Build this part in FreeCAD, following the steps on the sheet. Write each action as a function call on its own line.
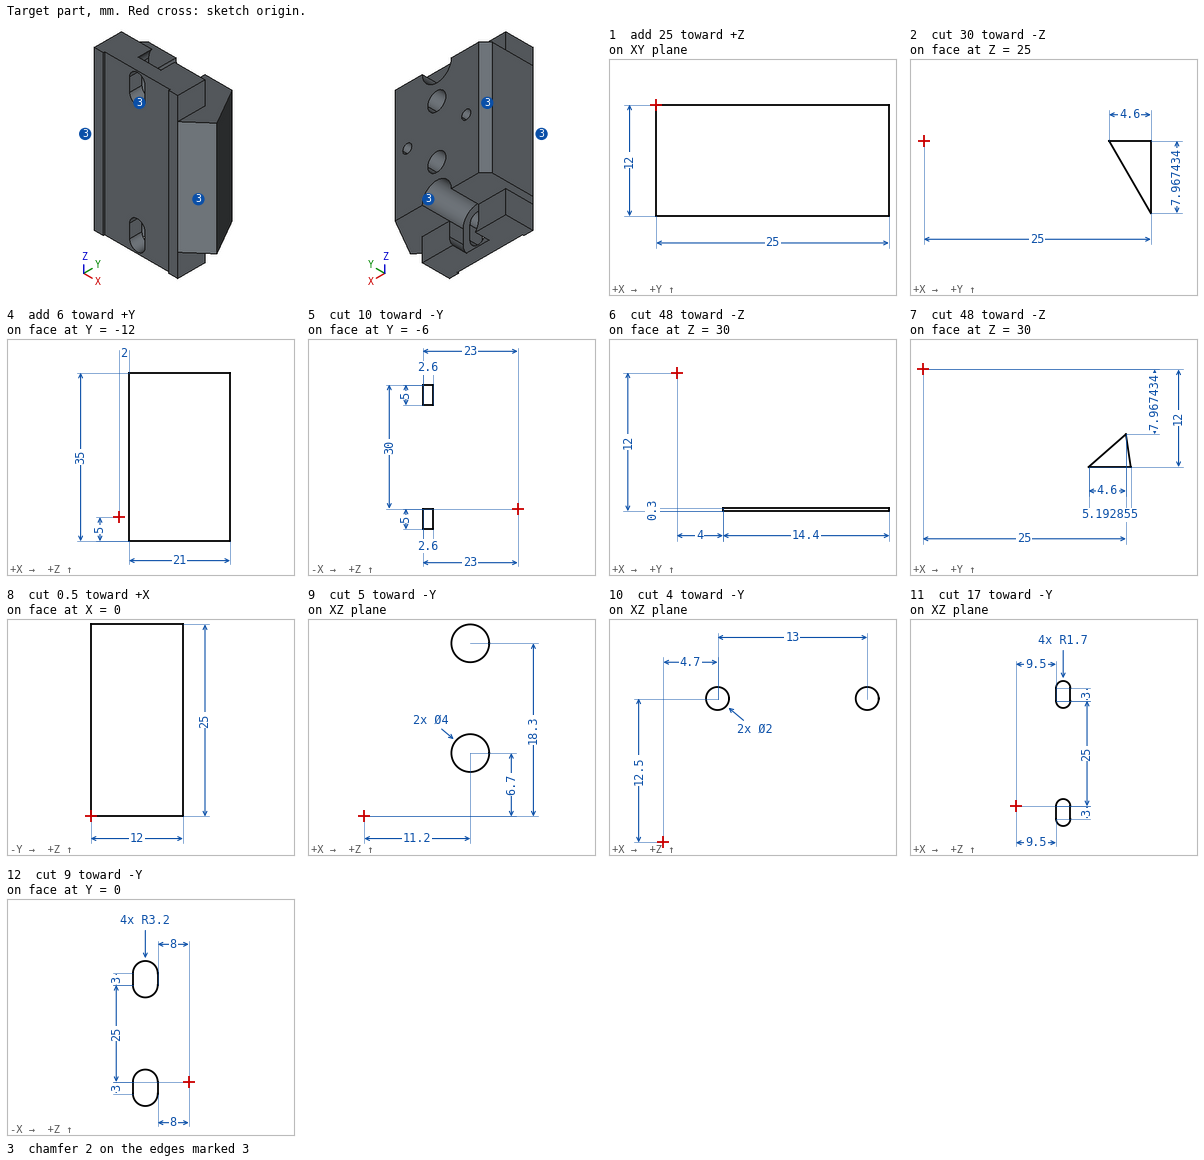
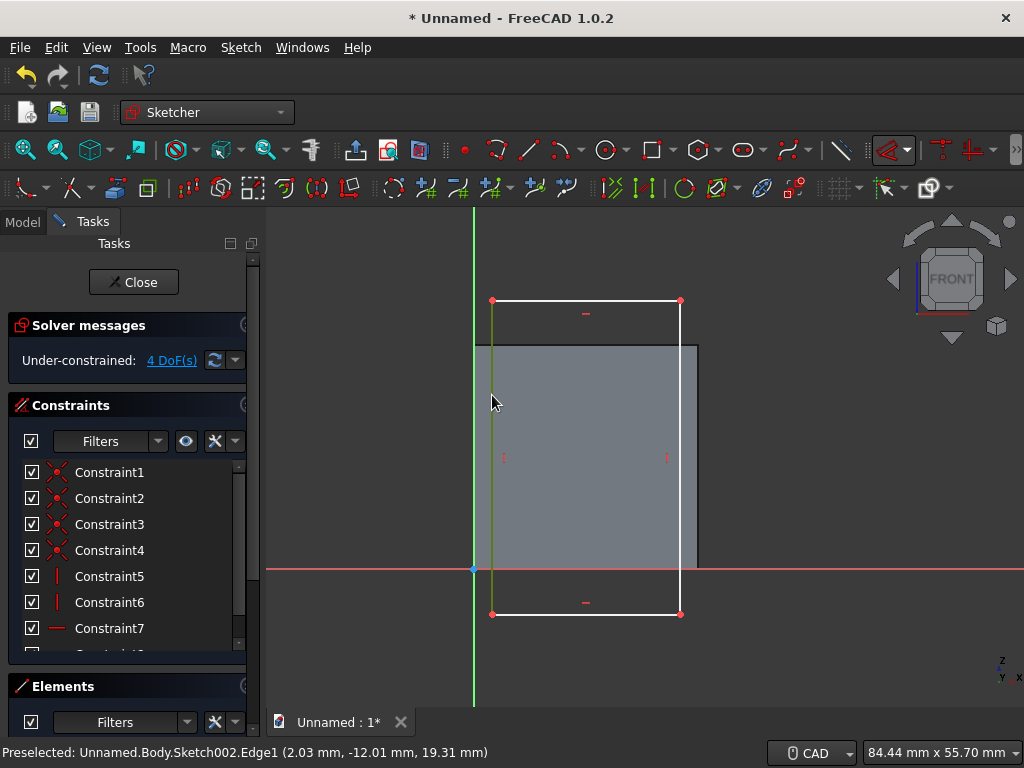
key(i)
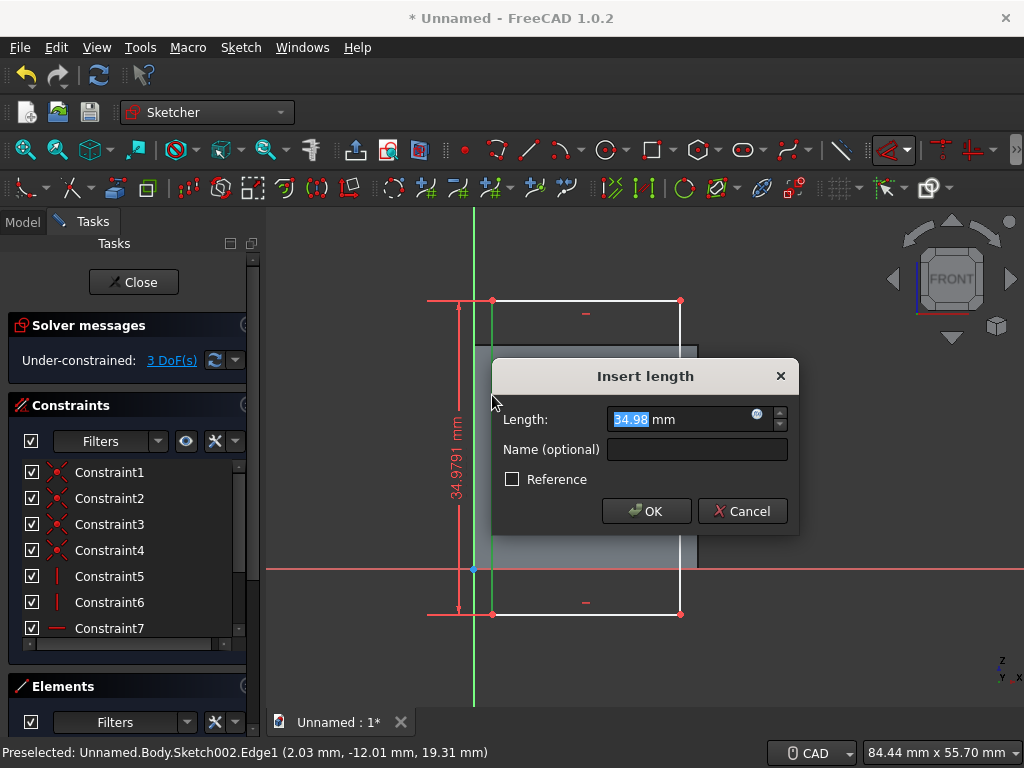
text(35)
key(Return)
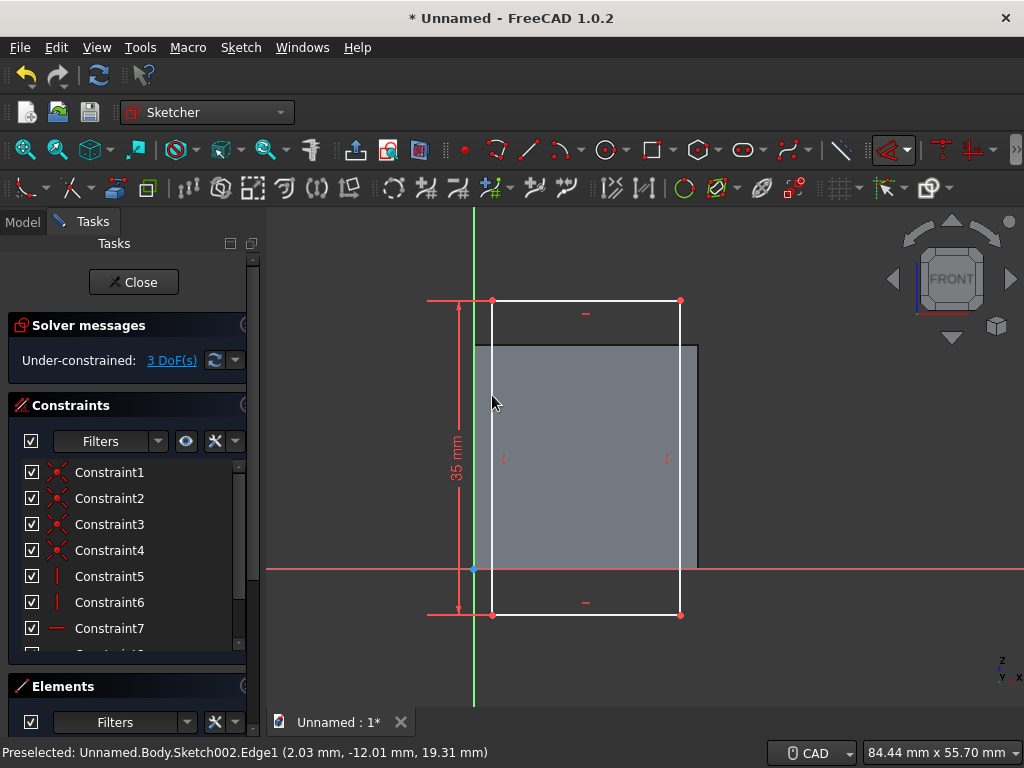
click(548, 615)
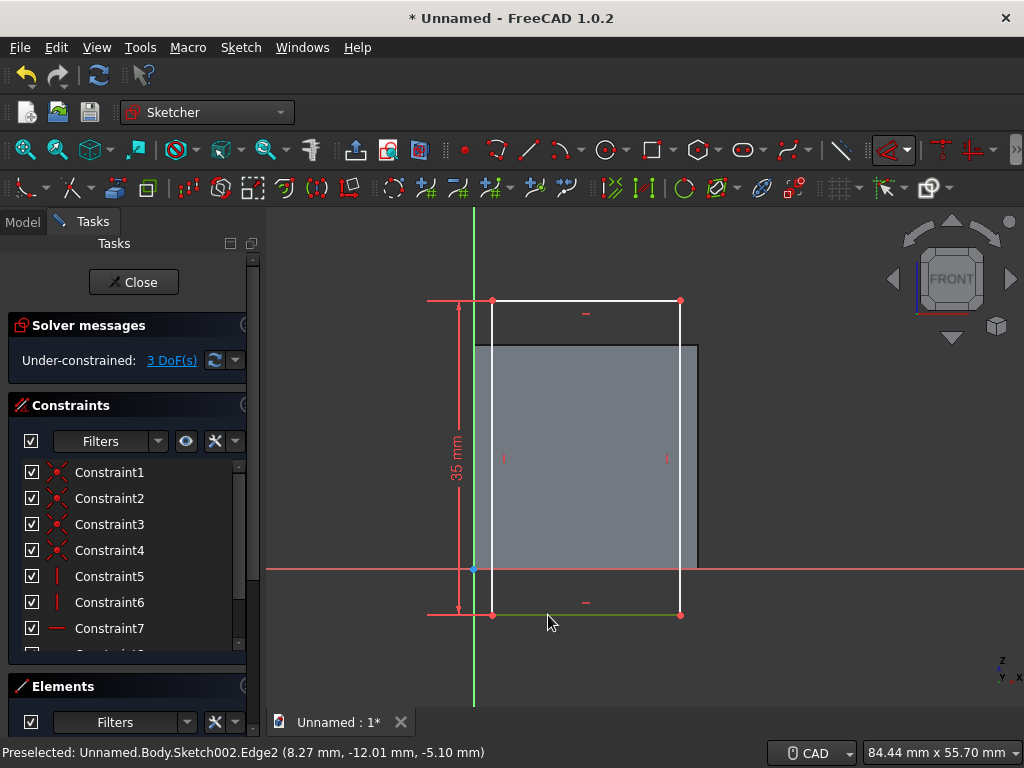
click(910, 150)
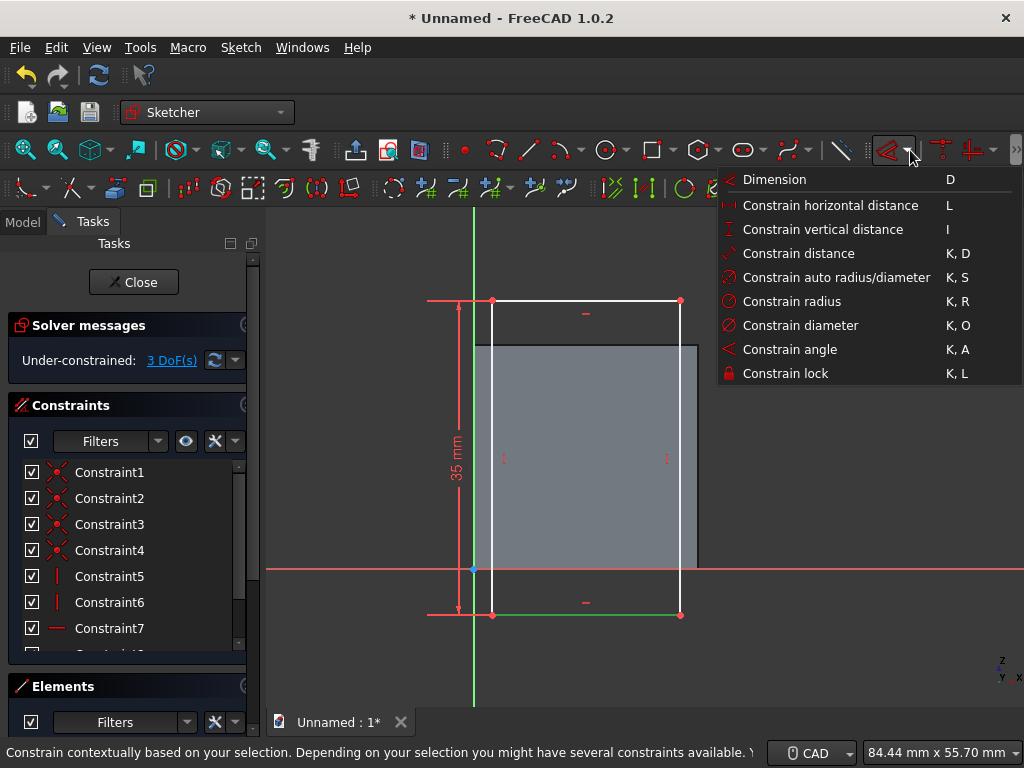
click(870, 205)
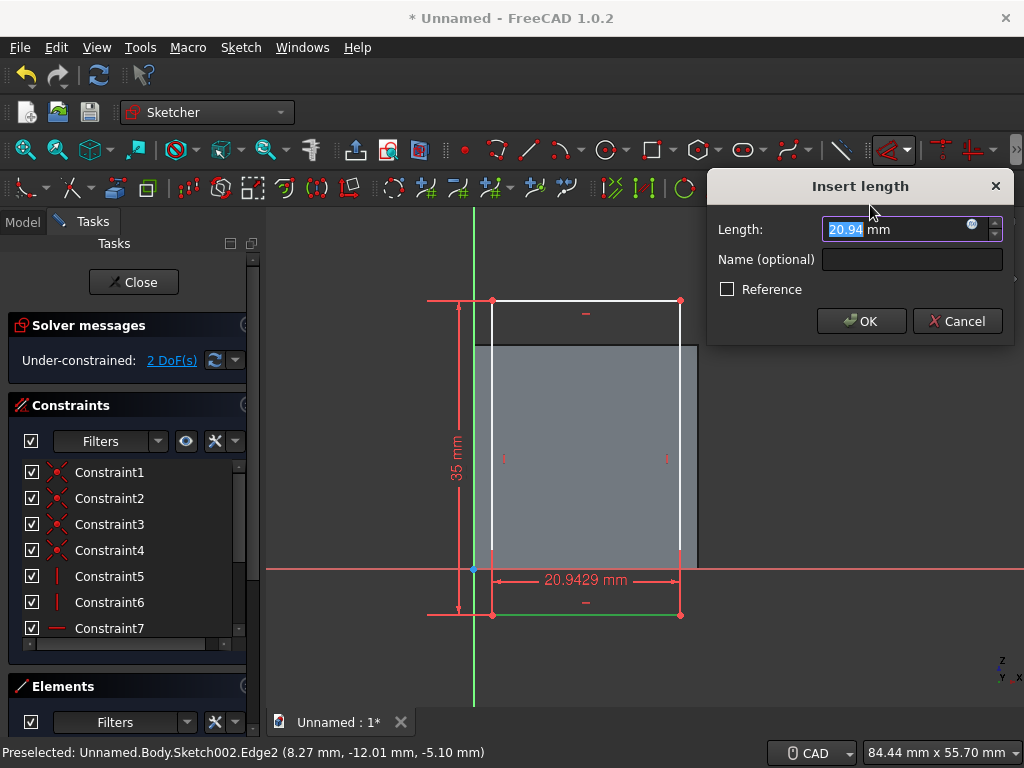
text(21)
key(Return)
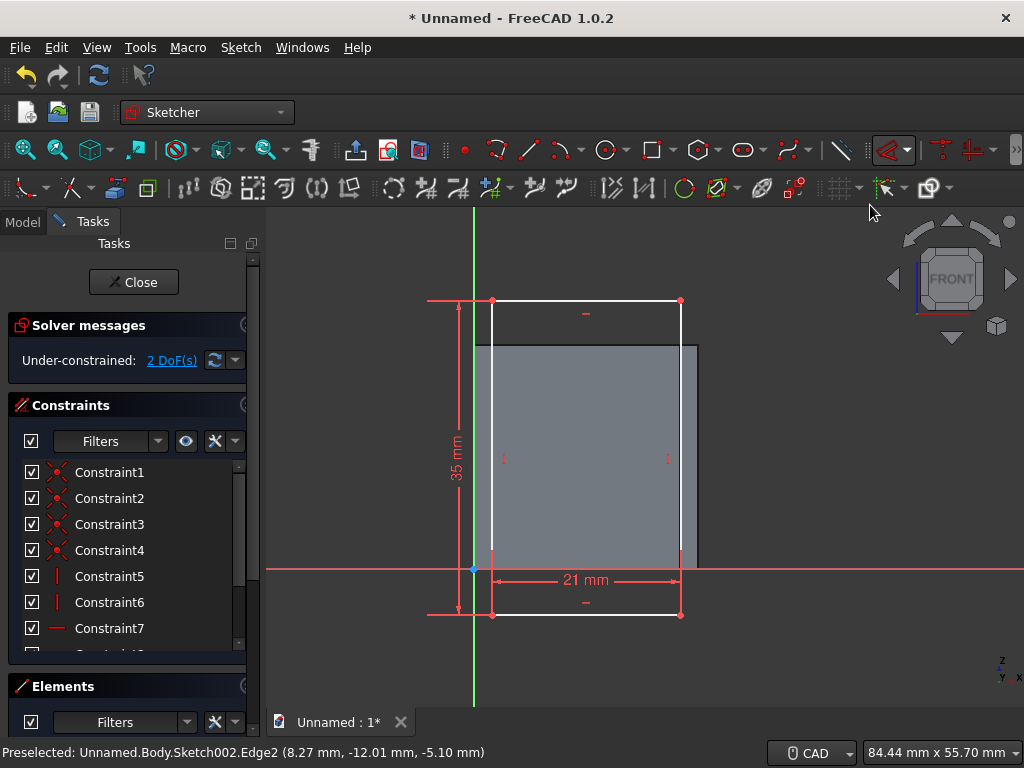
scroll(492, 301, up, 4)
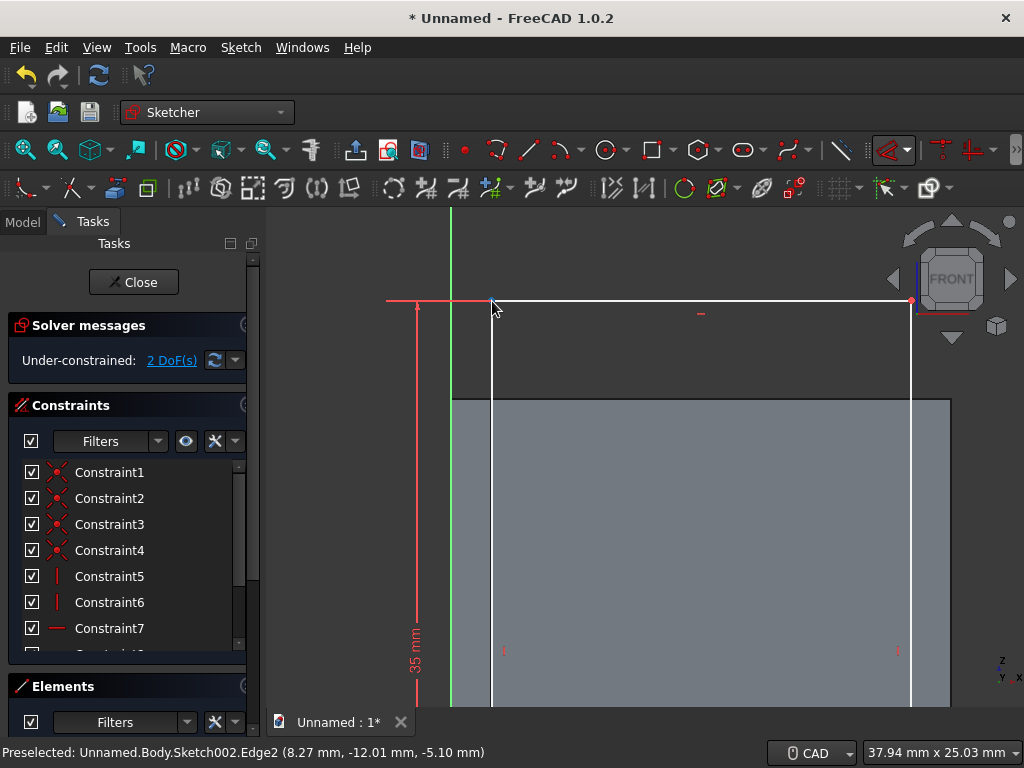
click(492, 301)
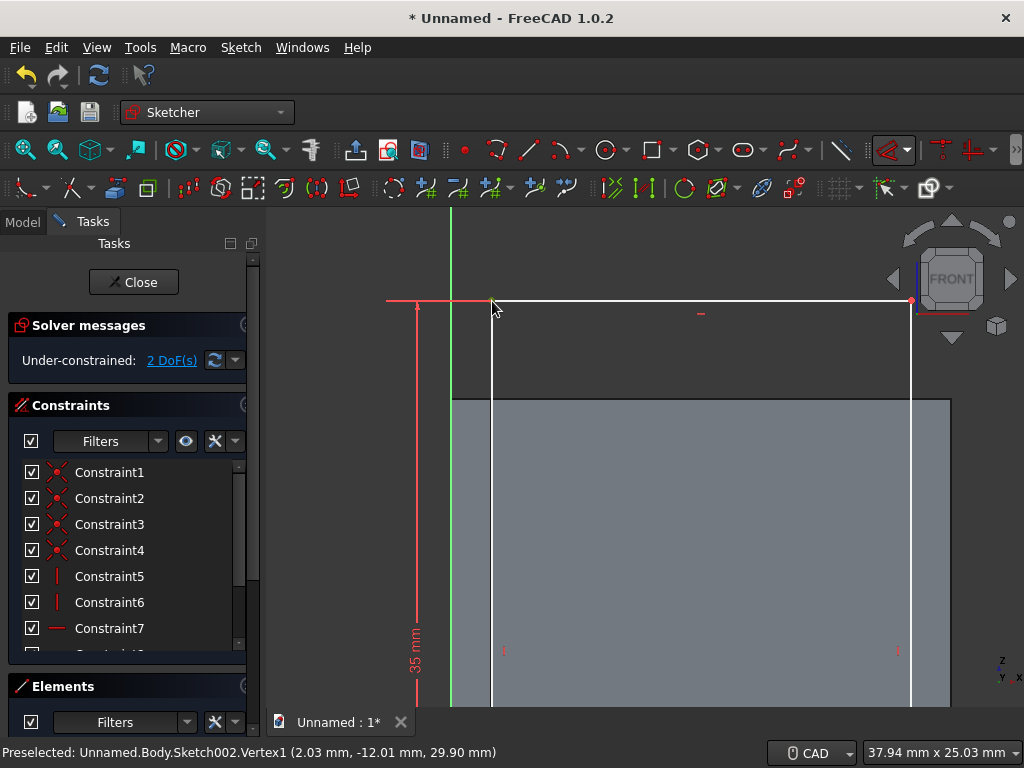
key(l)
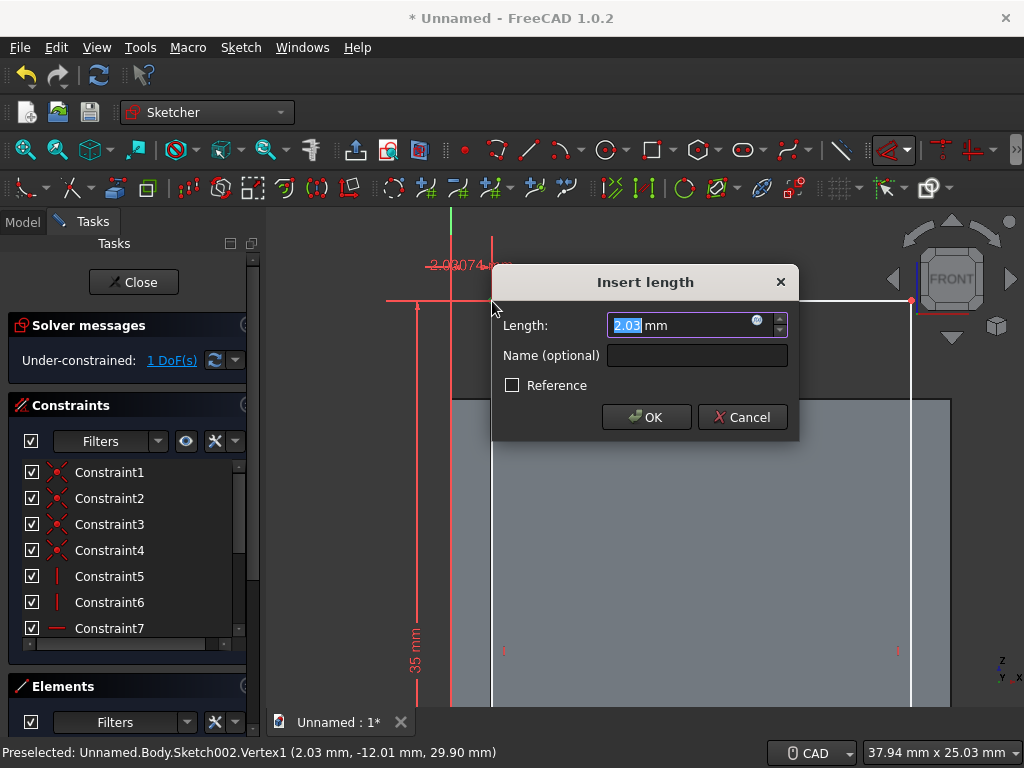
text(2)
key(Return)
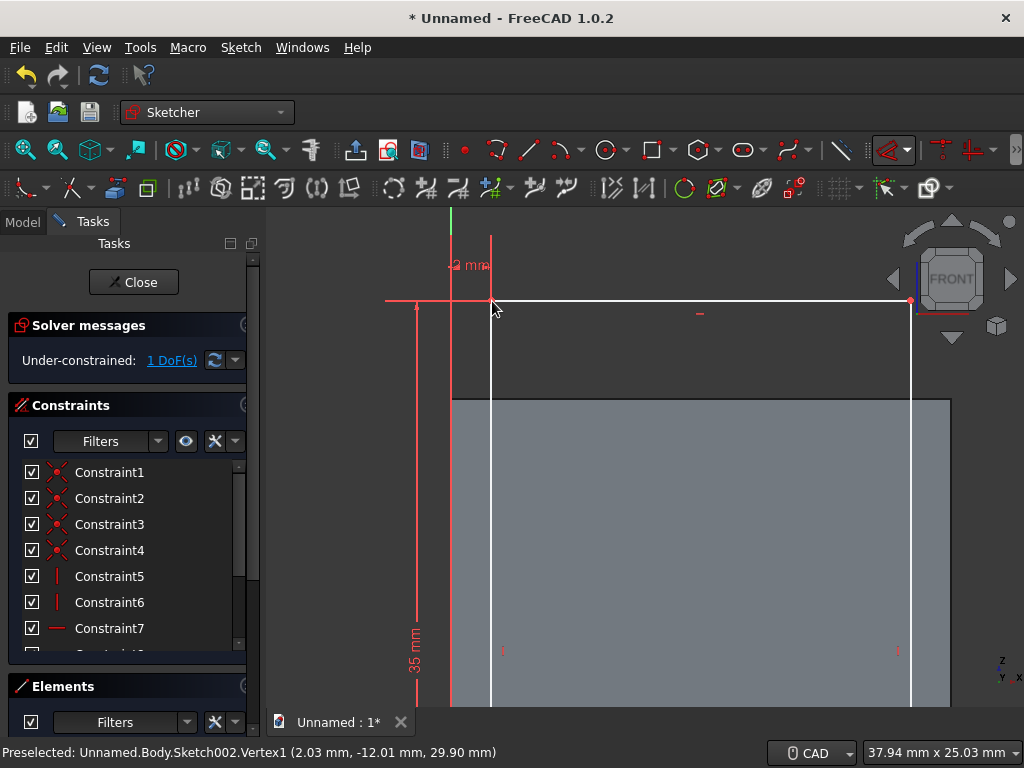
scroll(491, 301, down, 4)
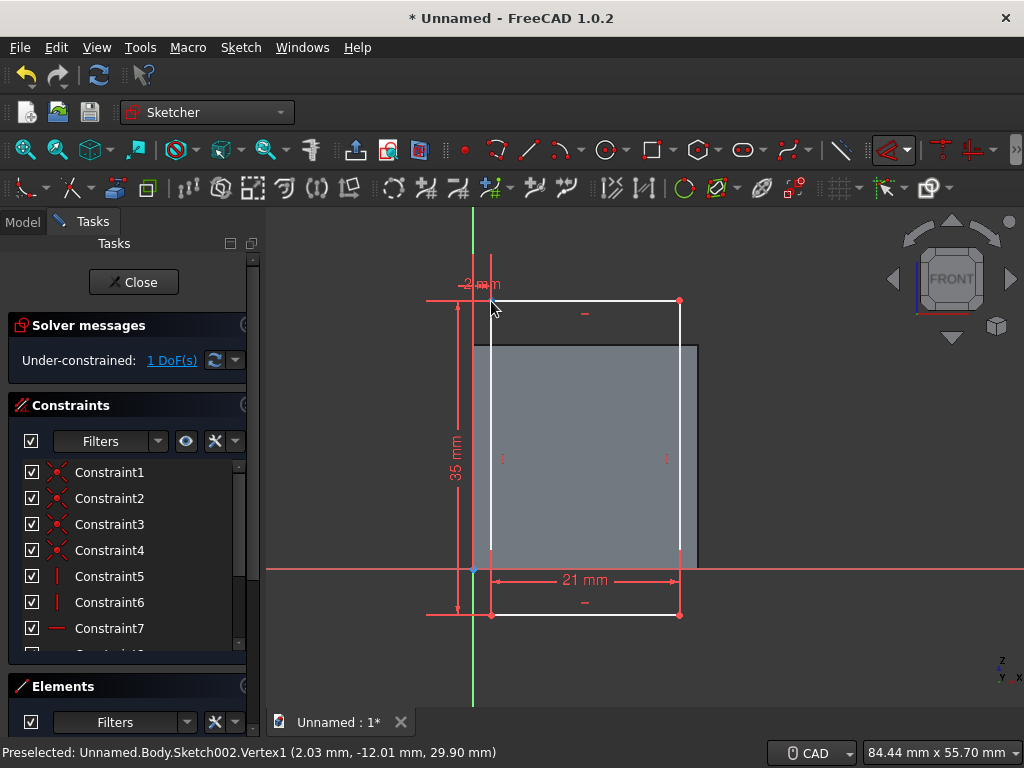
click(491, 615)